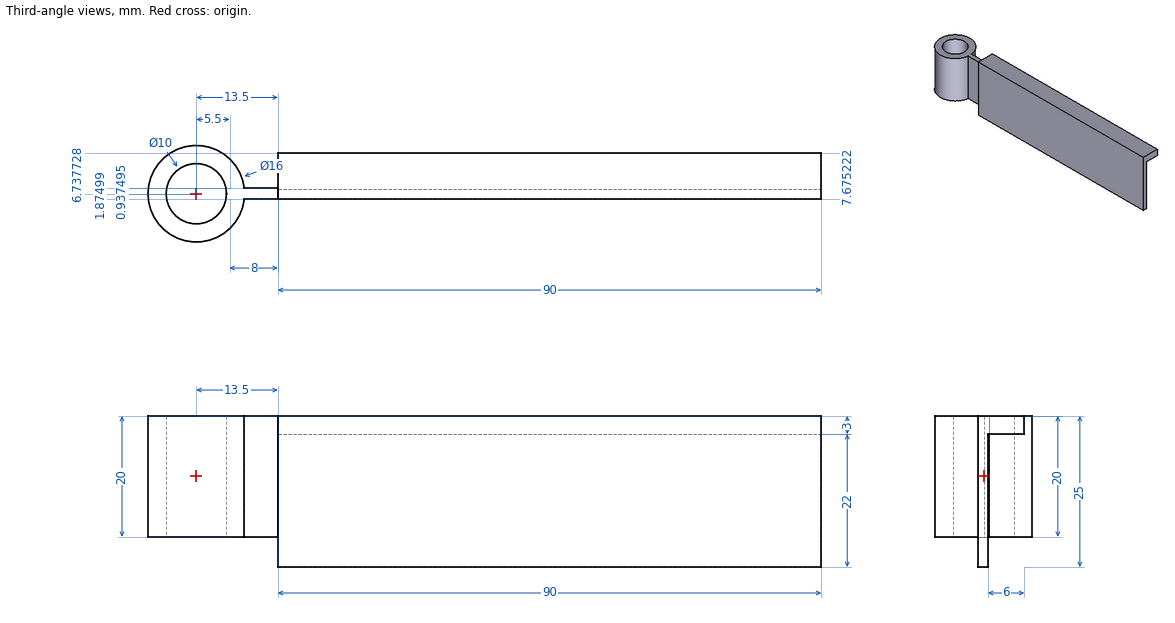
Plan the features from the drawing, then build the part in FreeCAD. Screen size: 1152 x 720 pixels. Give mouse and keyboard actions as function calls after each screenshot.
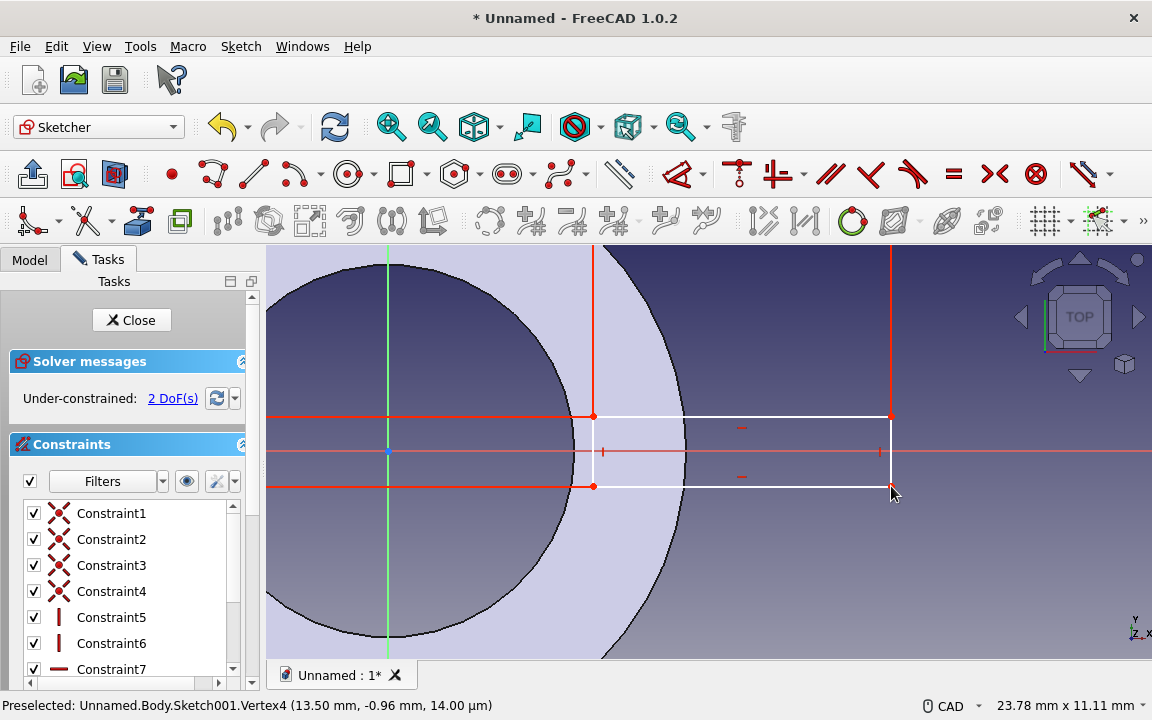
click(593, 417)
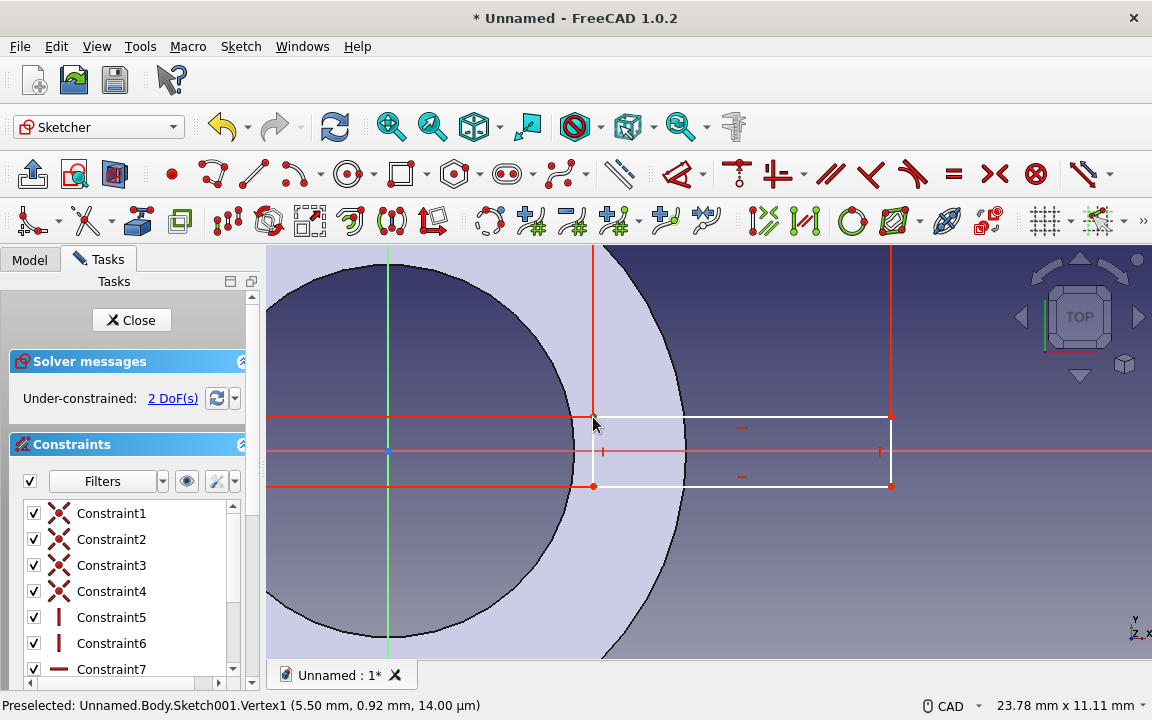
click(702, 174)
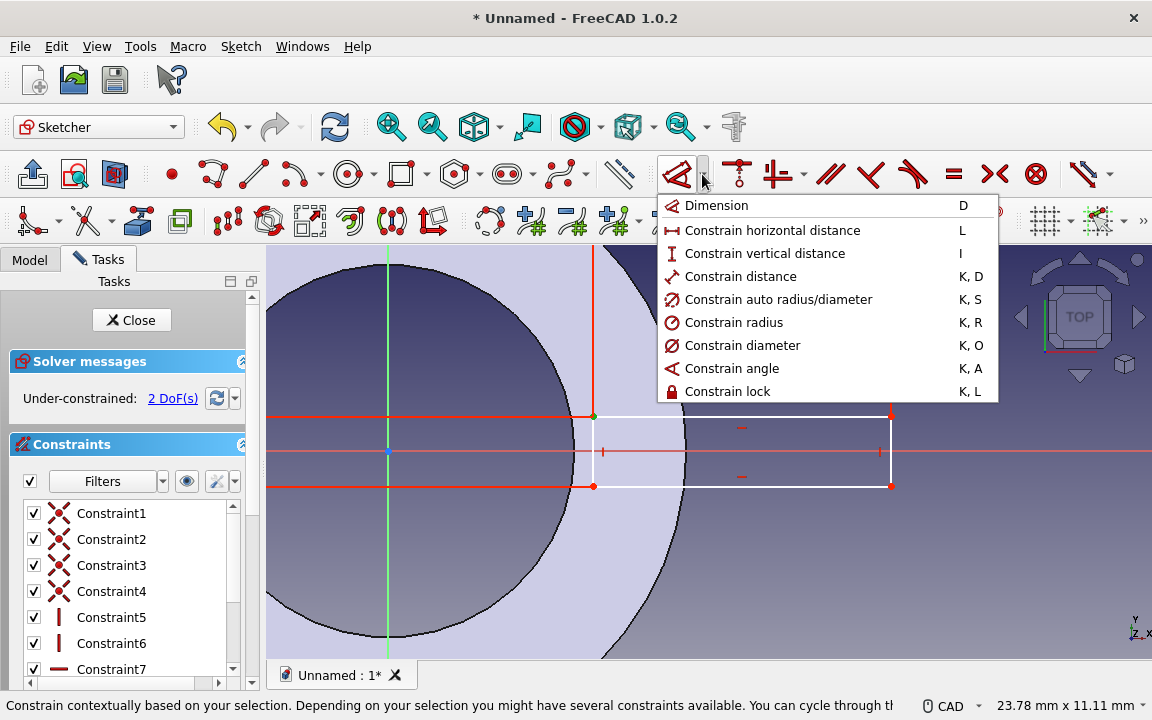
click(828, 230)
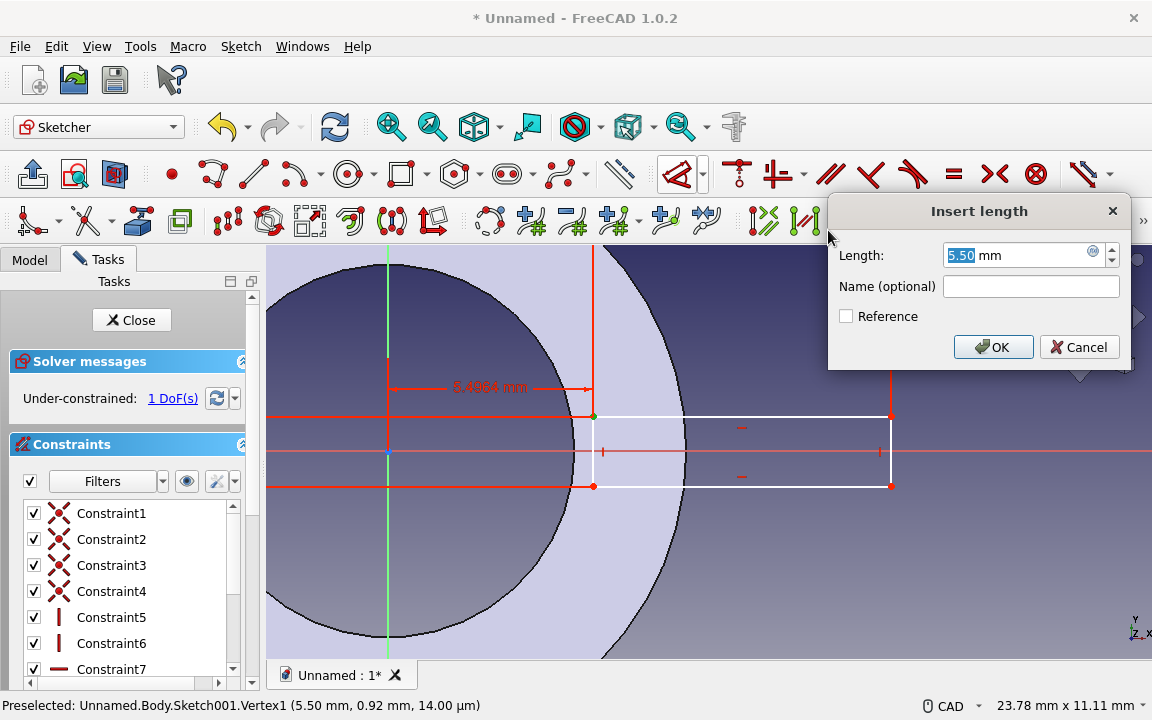
text(5.5)
key(Return)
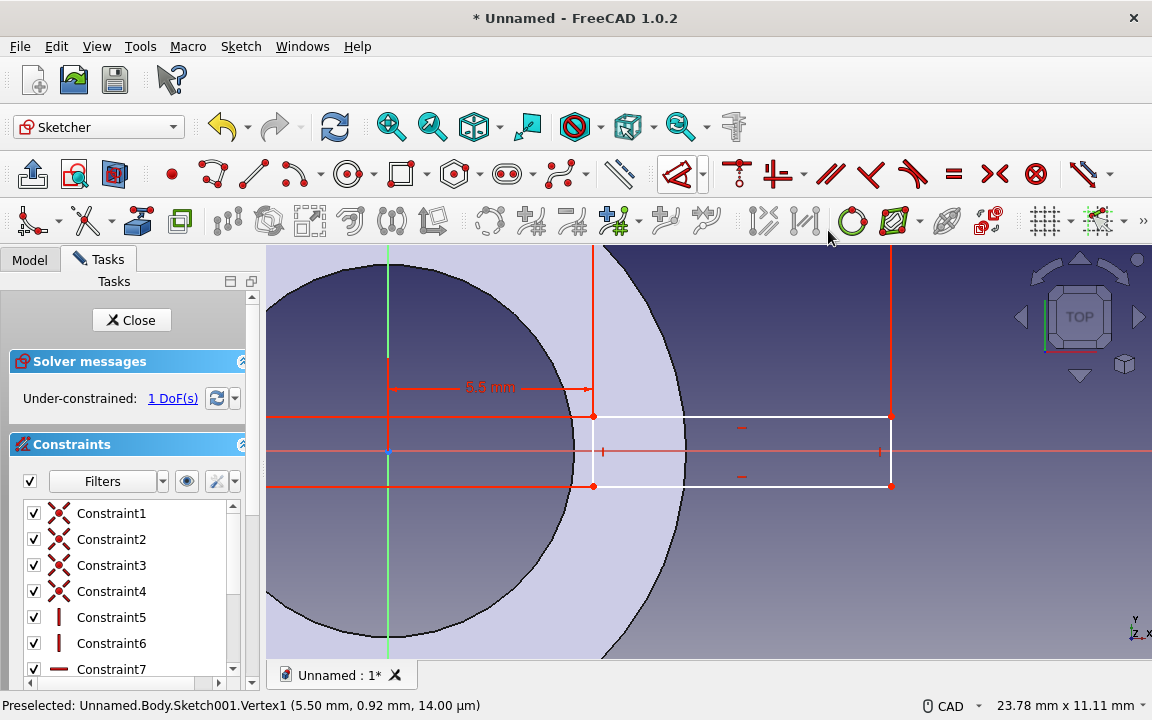
click(593, 417)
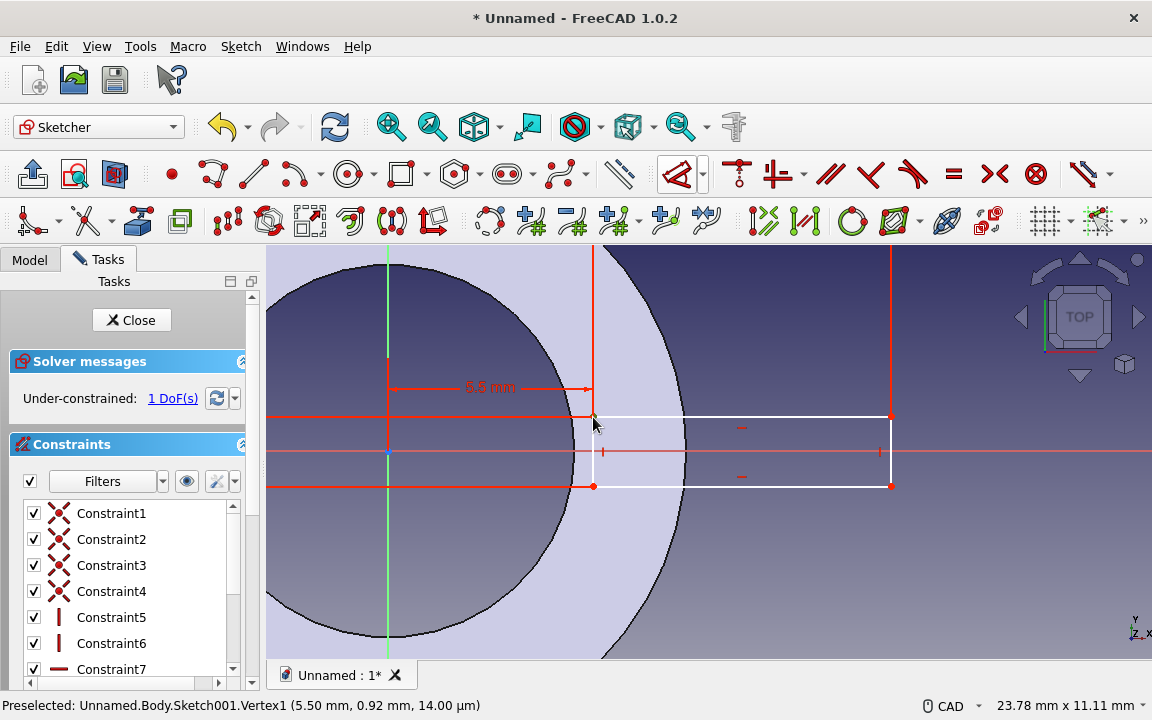
click(702, 174)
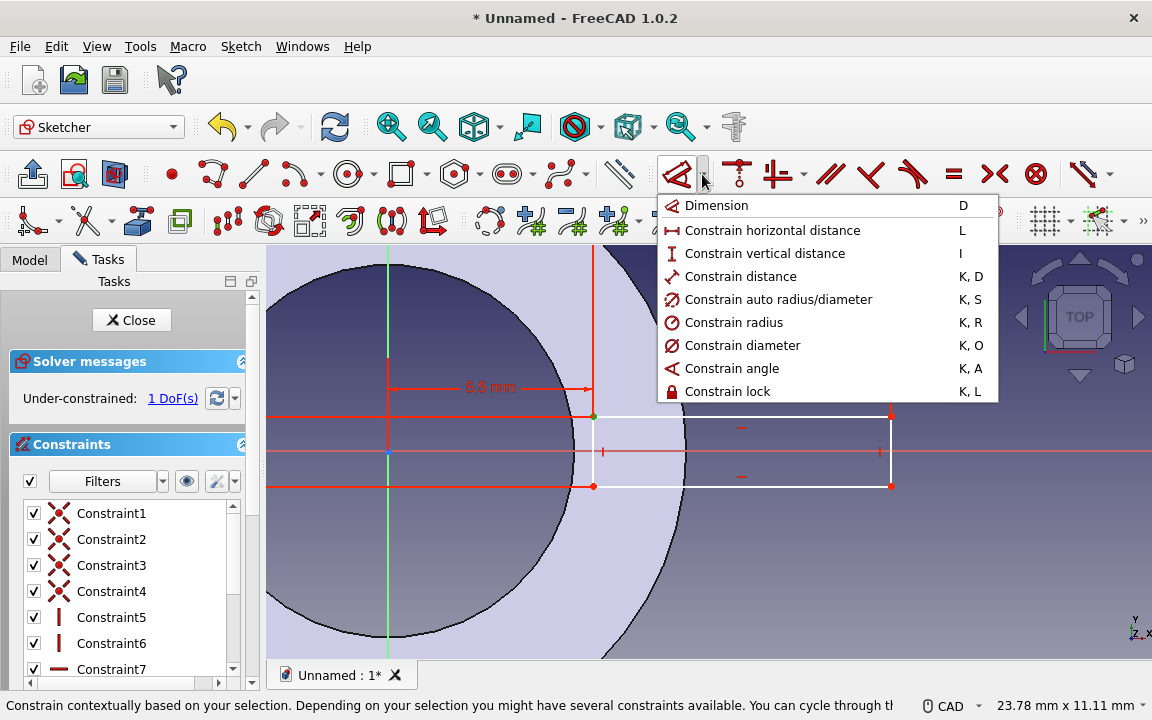
click(828, 254)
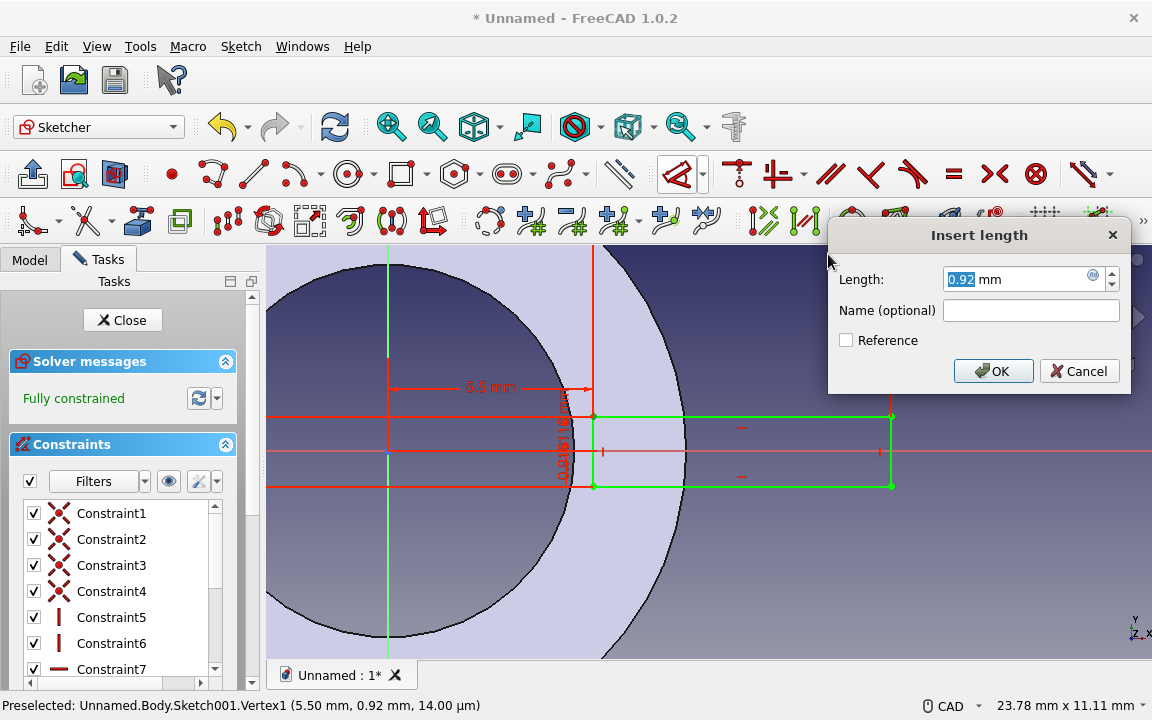
text(0.937495)
key(Return)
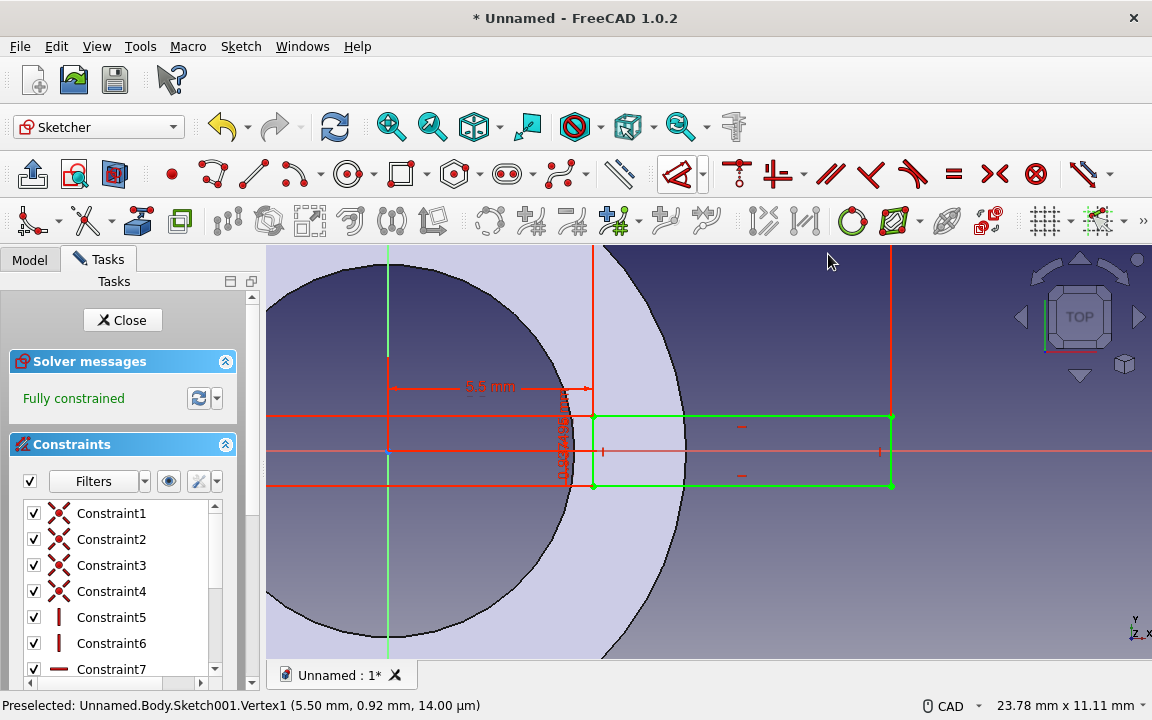
click(123, 320)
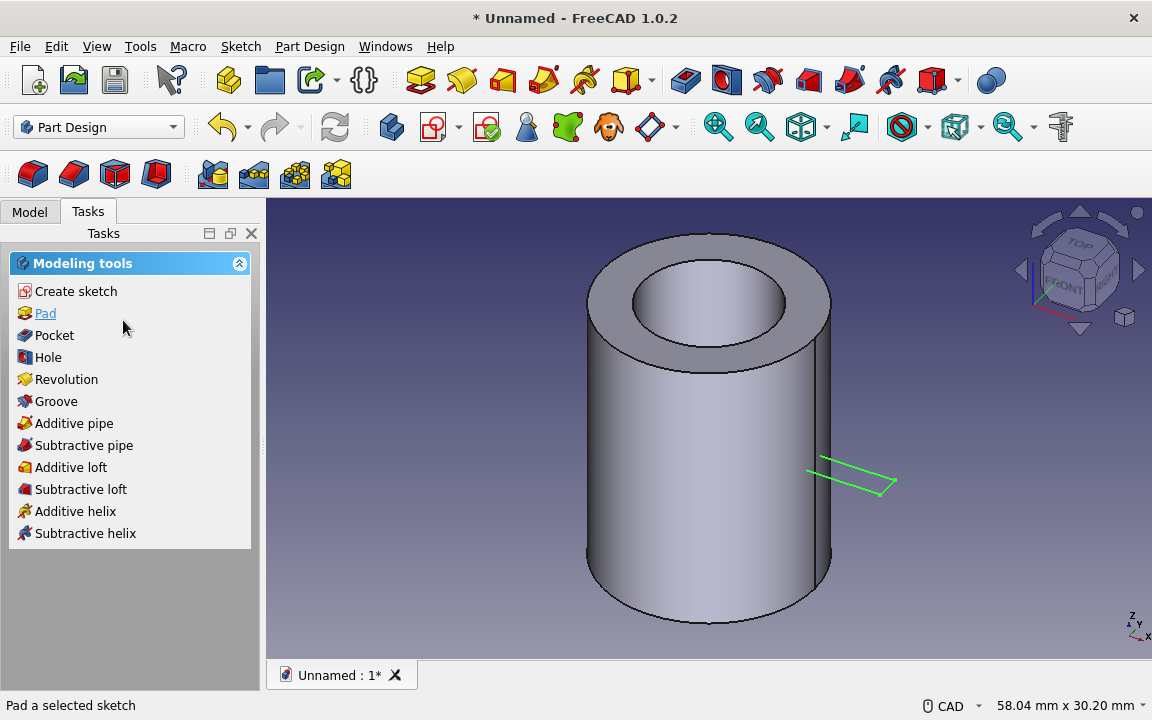
click(421, 80)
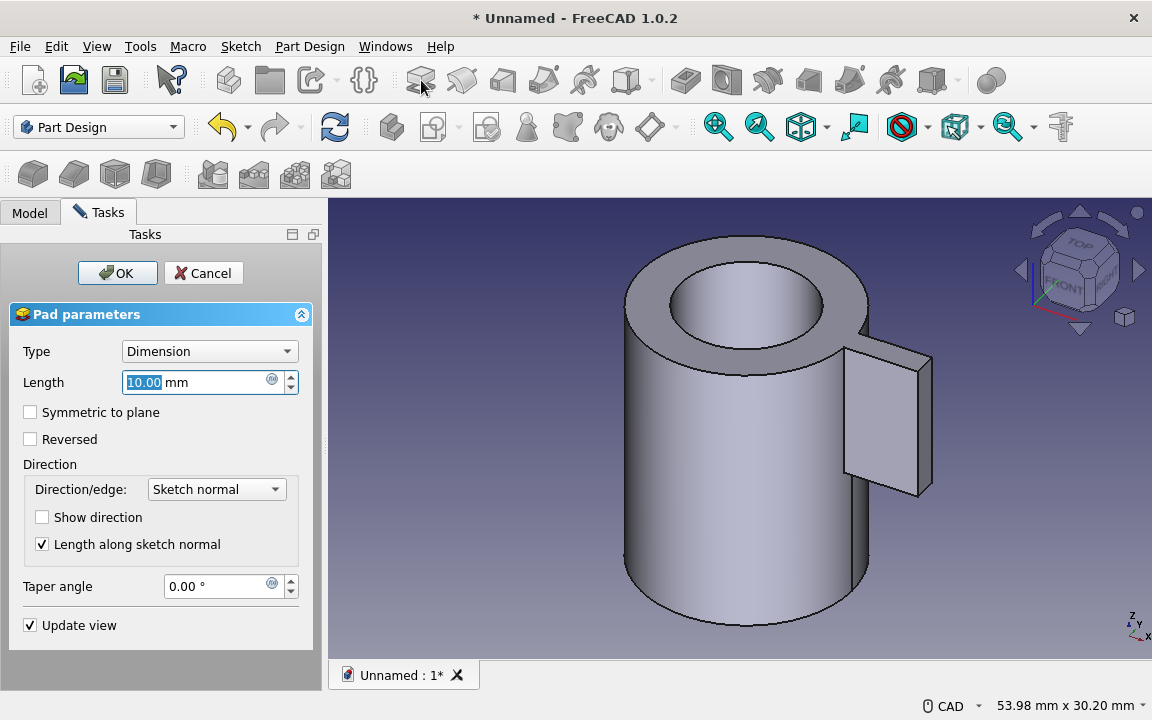
text(20)
key(Tab)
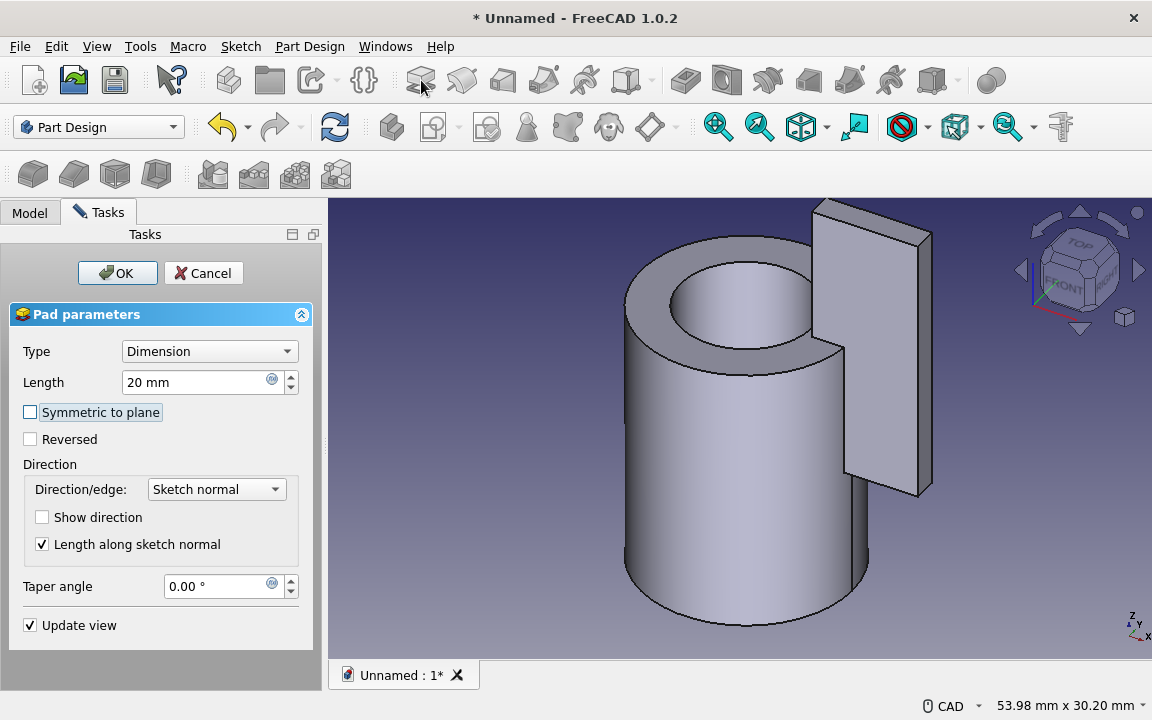
click(31, 412)